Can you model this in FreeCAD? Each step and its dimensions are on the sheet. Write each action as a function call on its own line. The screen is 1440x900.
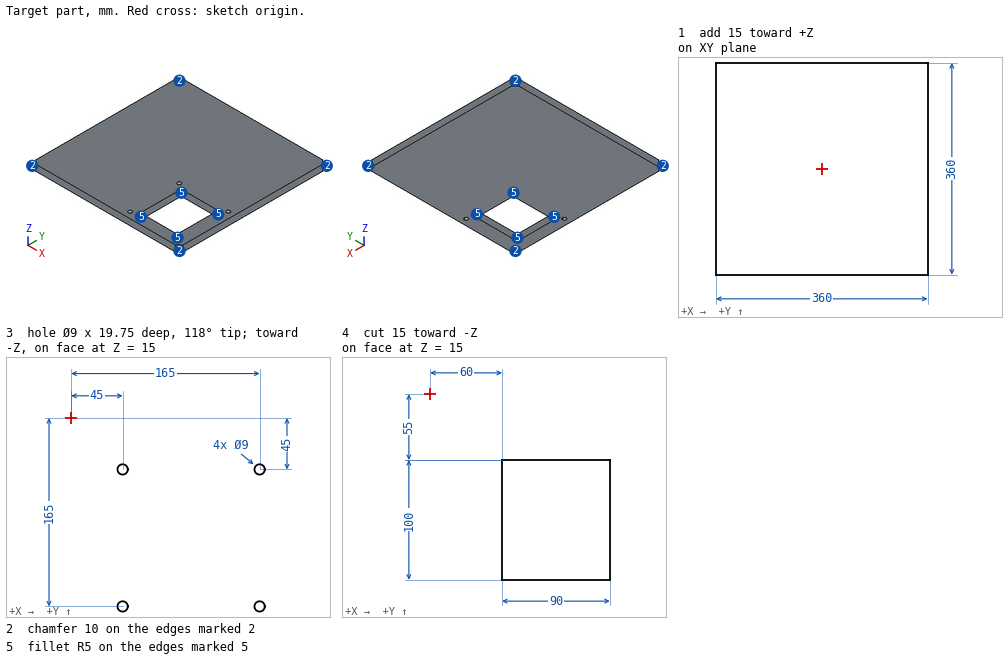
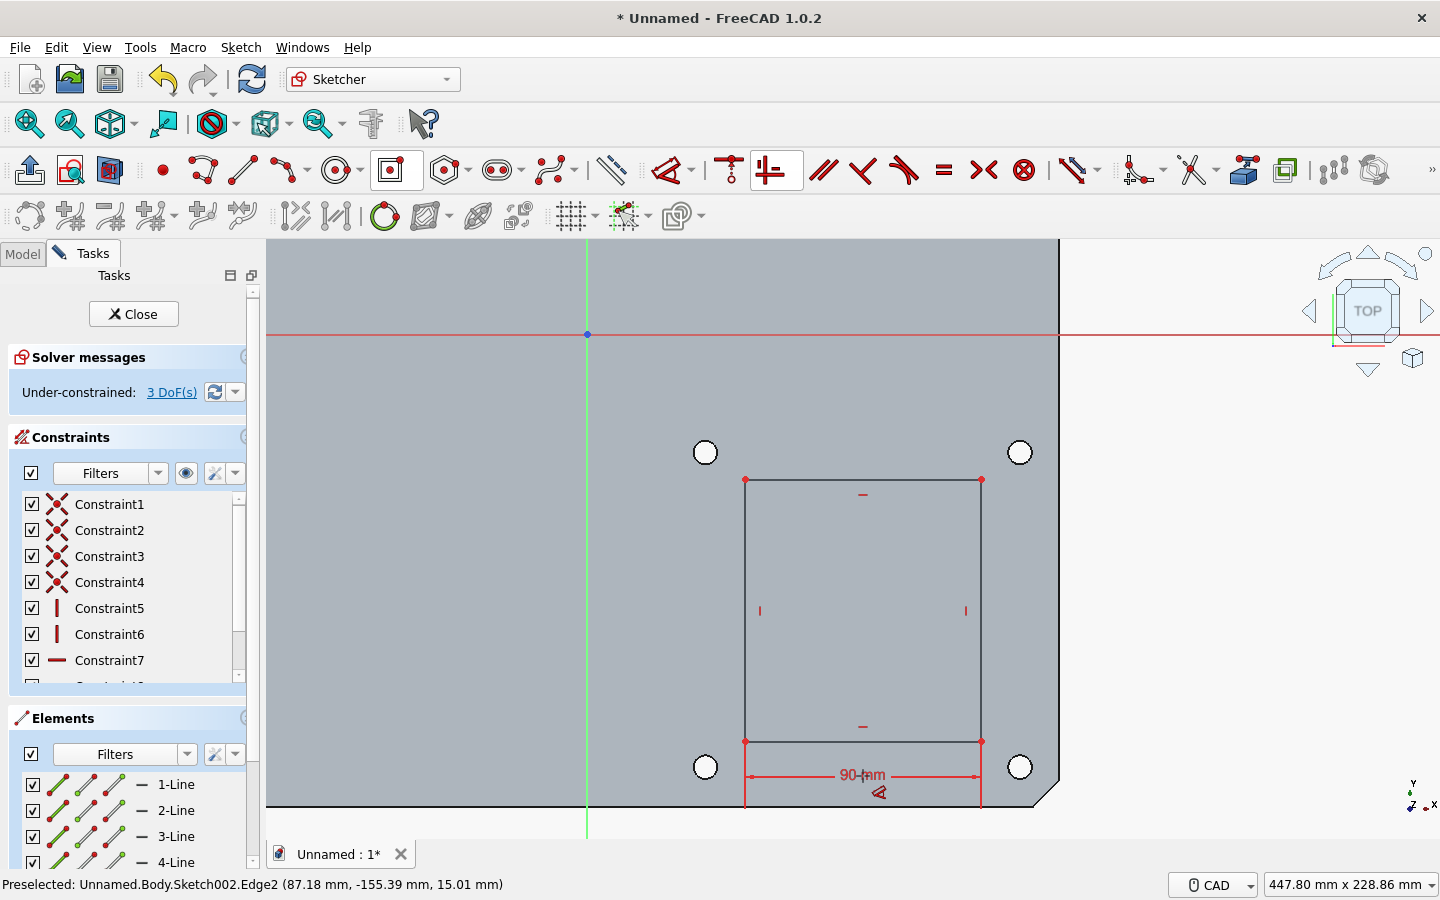
click(745, 559)
click(711, 611)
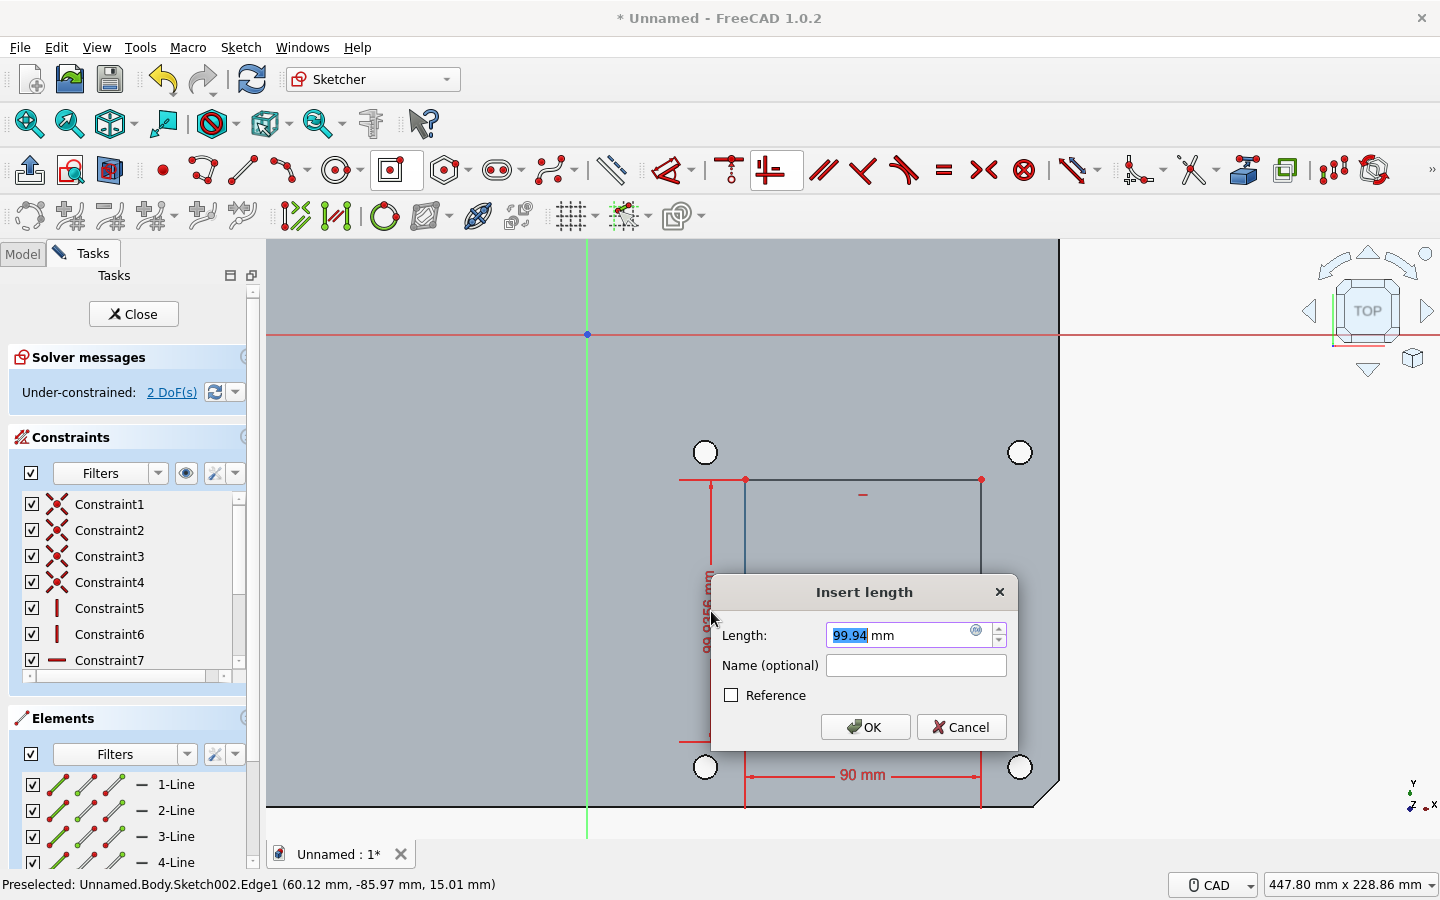
text(100)
key(Return)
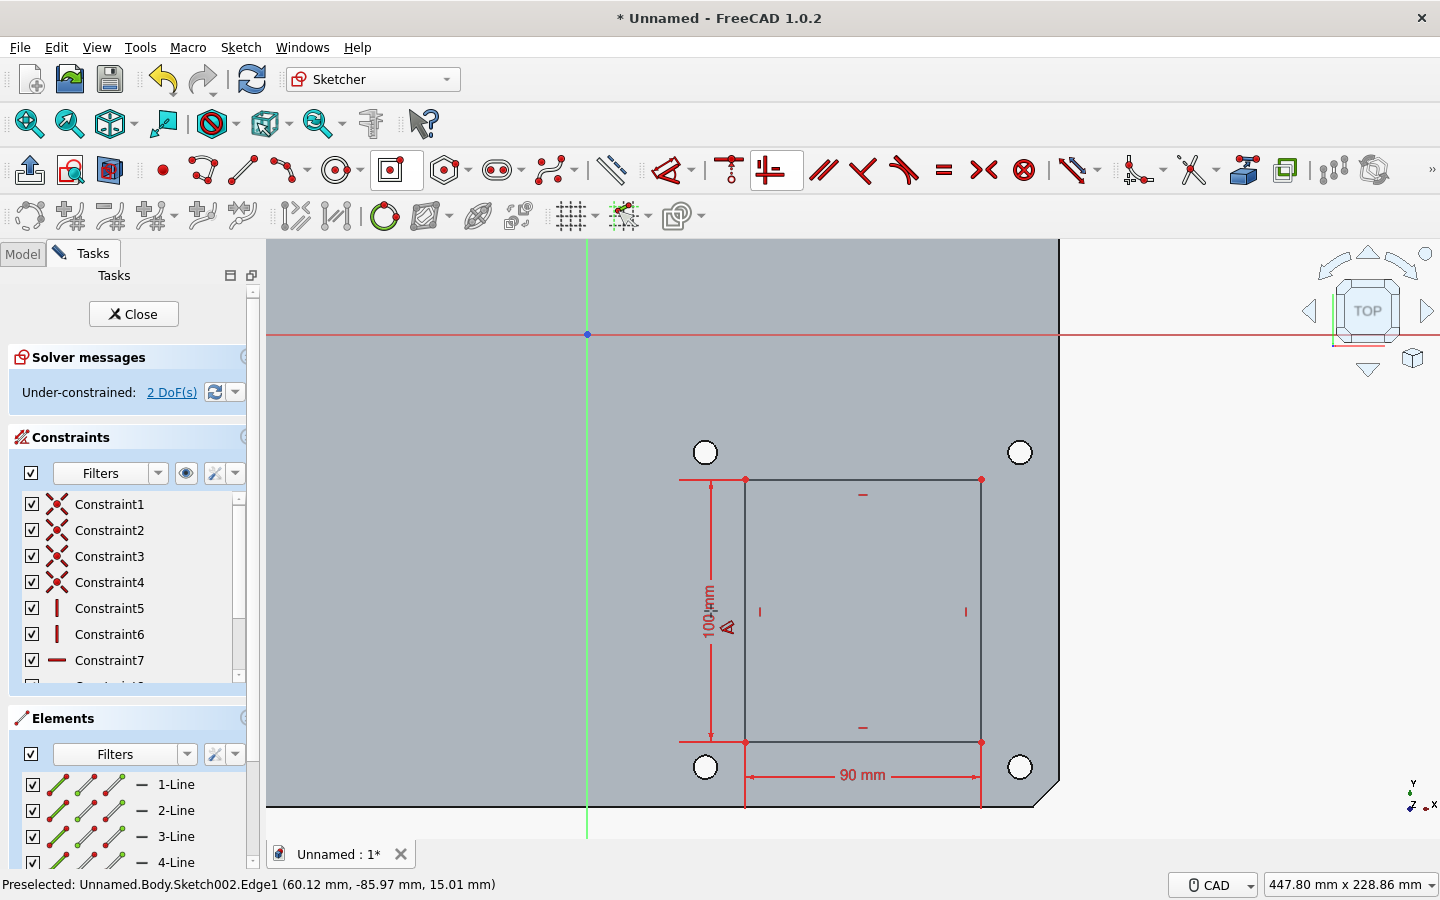
click(745, 480)
click(666, 301)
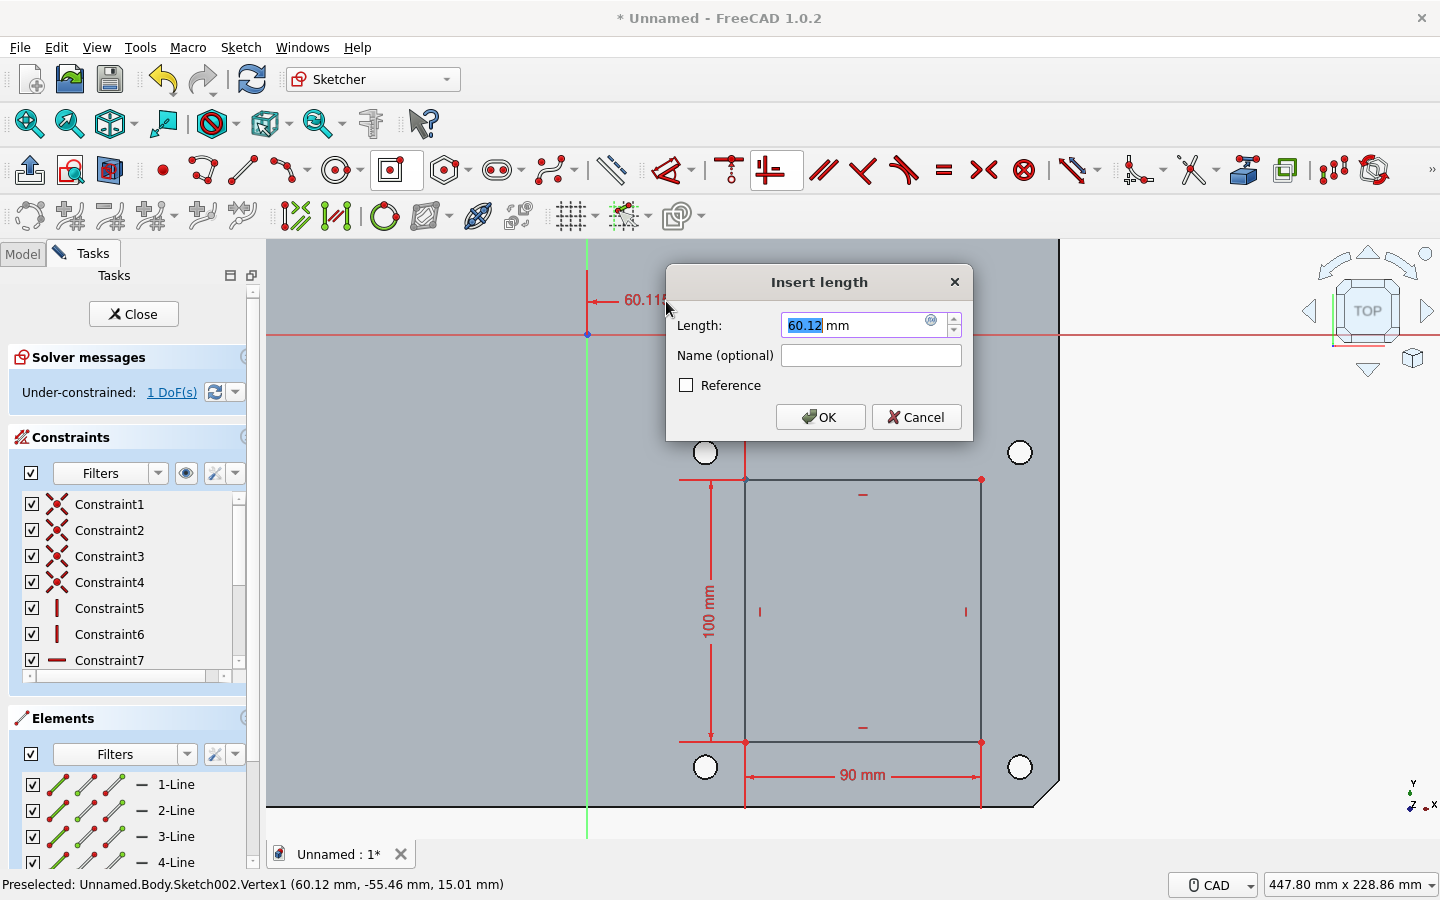
text(60)
key(Return)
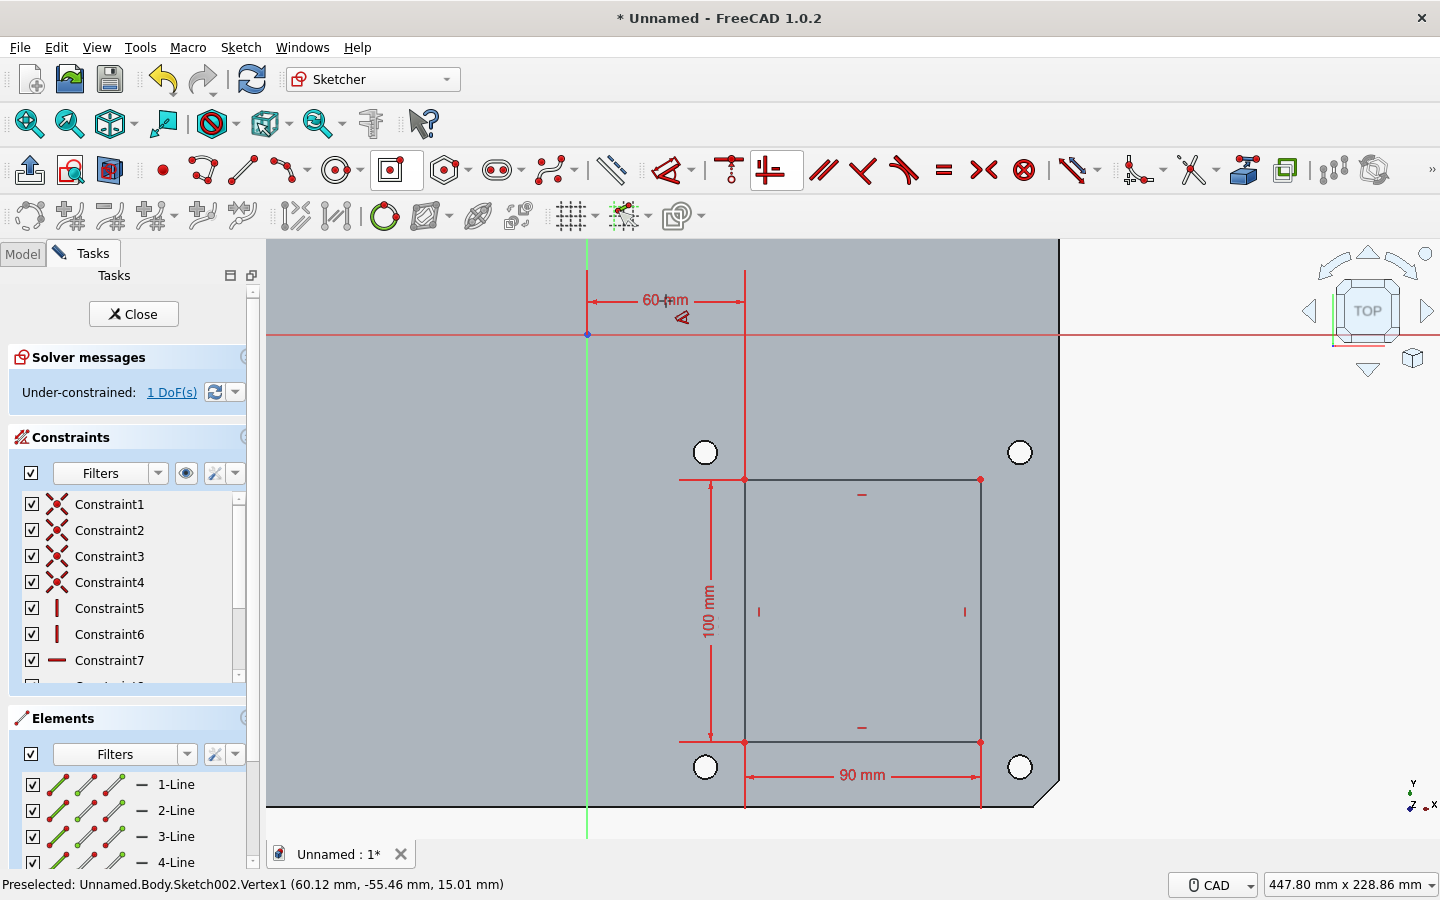
click(745, 480)
click(553, 407)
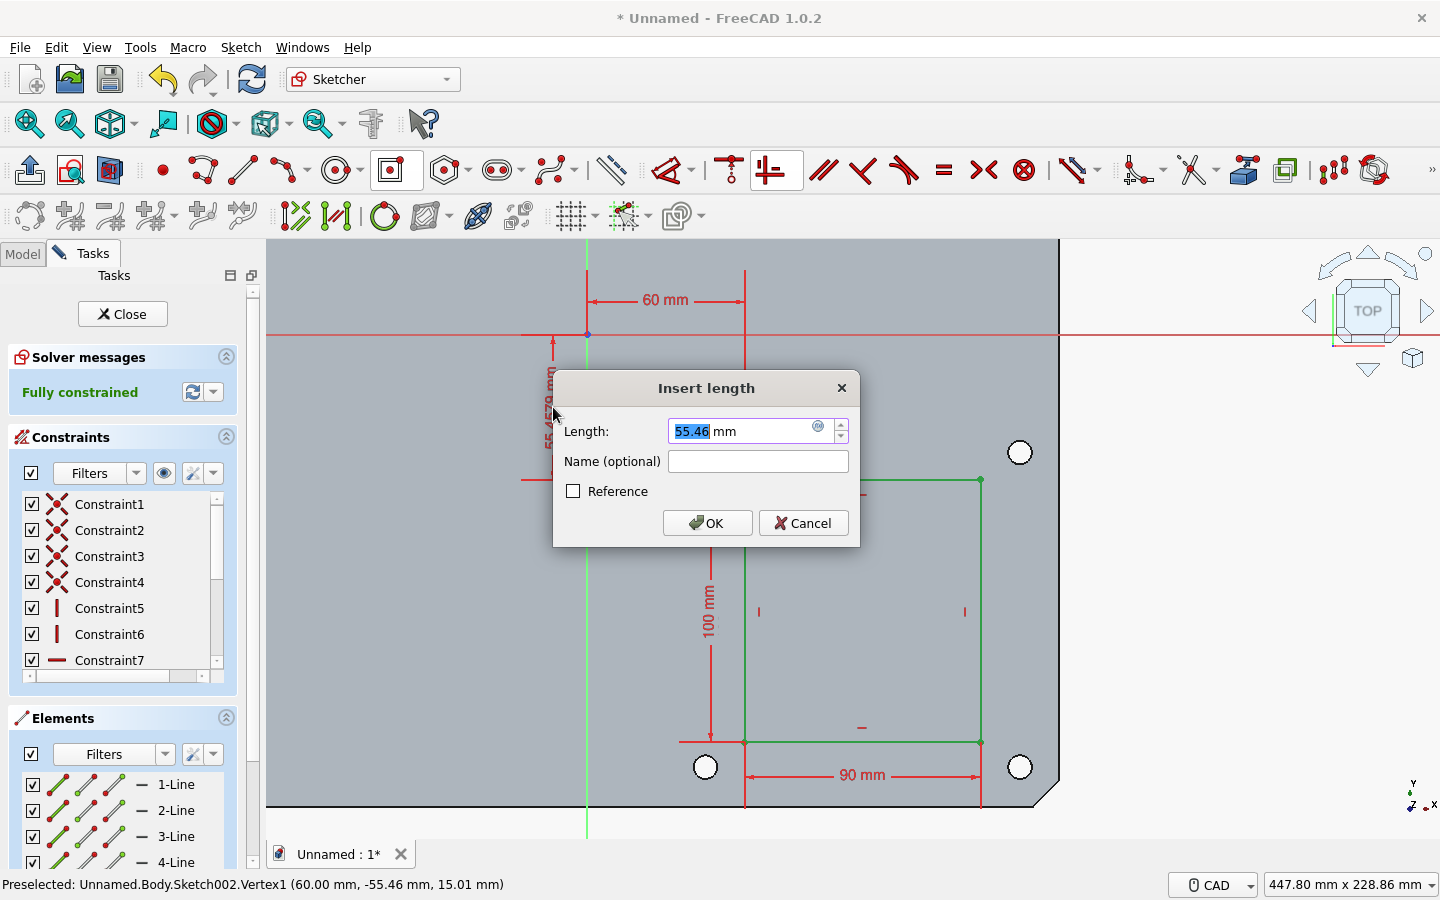
text(55)
key(Return)
key(Escape)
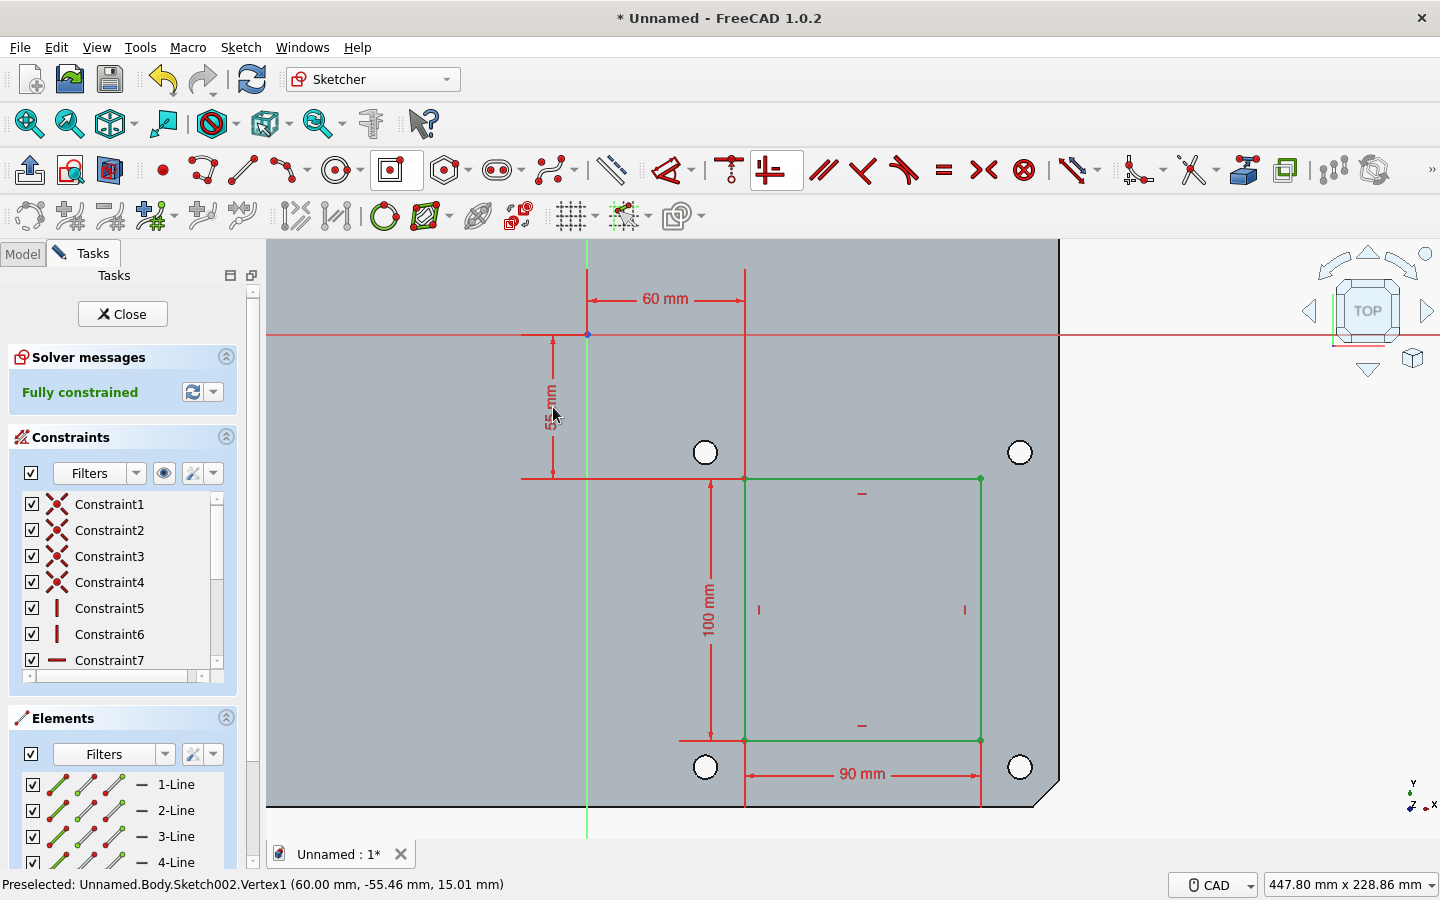
click(123, 314)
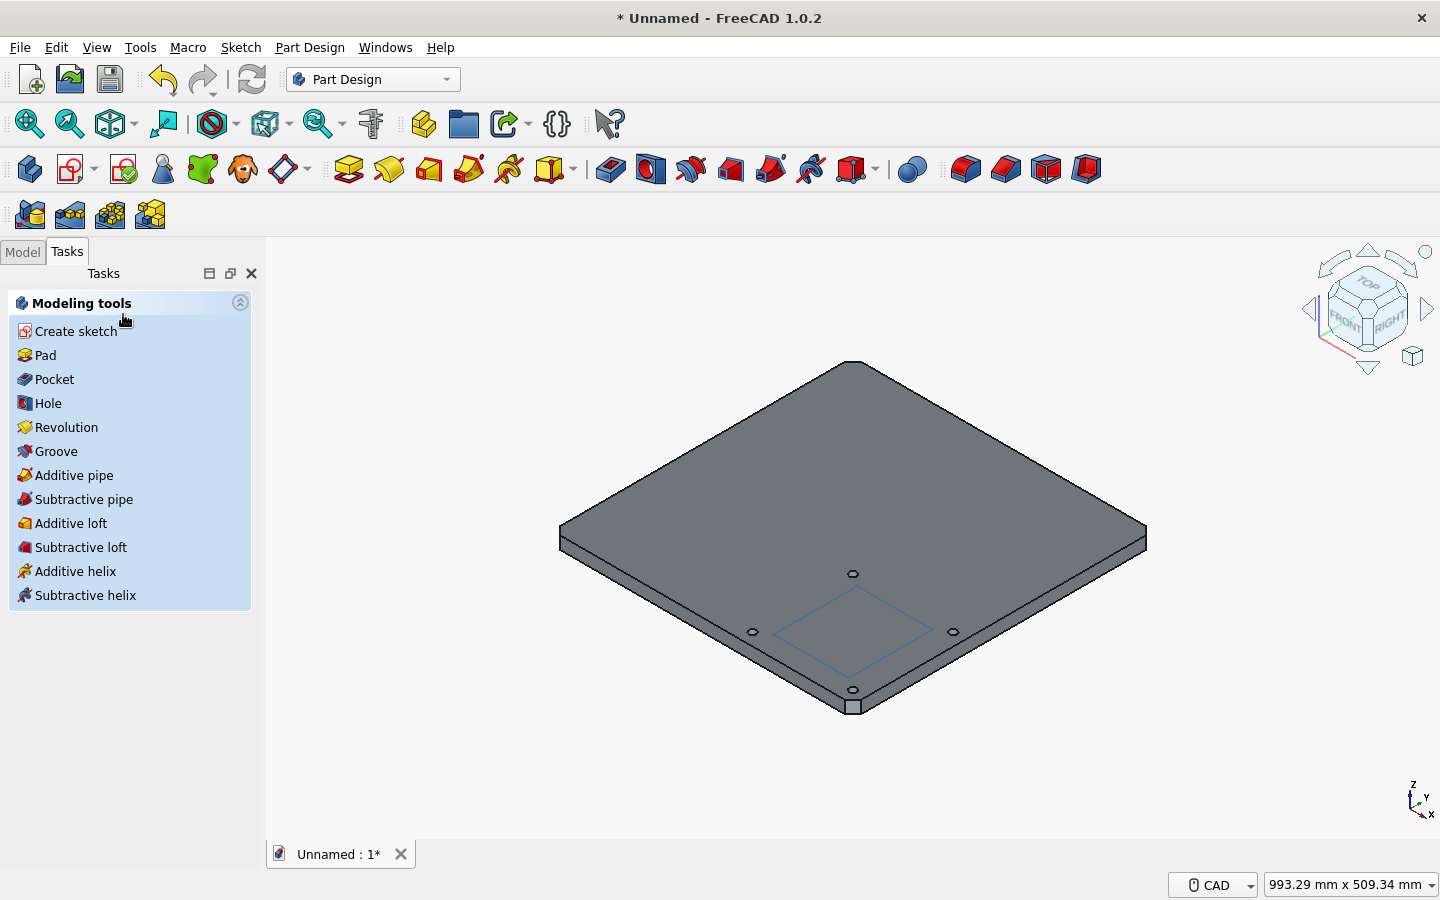
click(612, 170)